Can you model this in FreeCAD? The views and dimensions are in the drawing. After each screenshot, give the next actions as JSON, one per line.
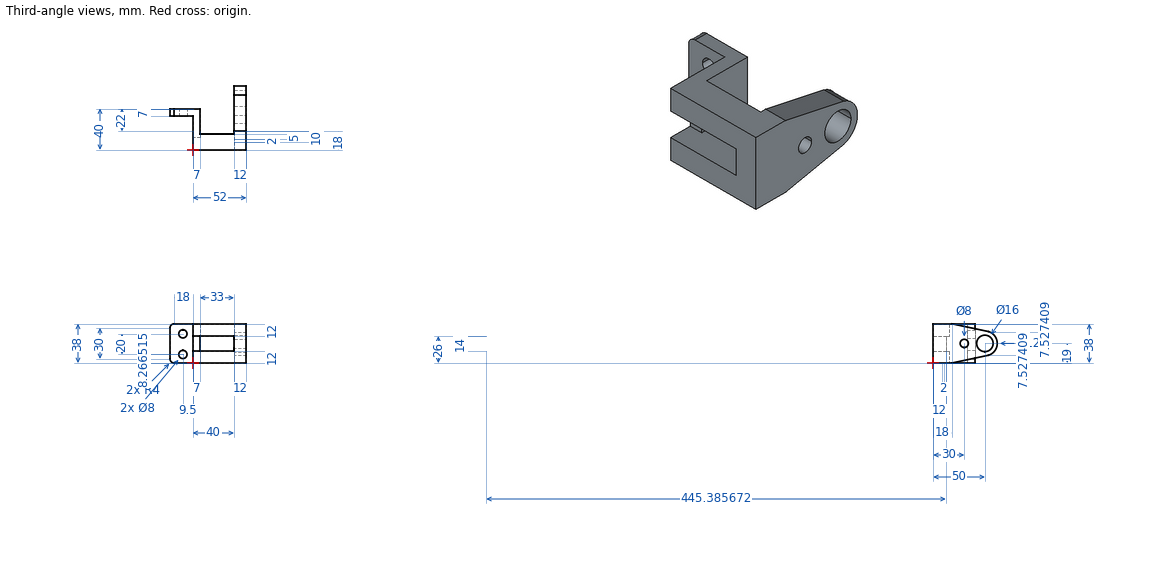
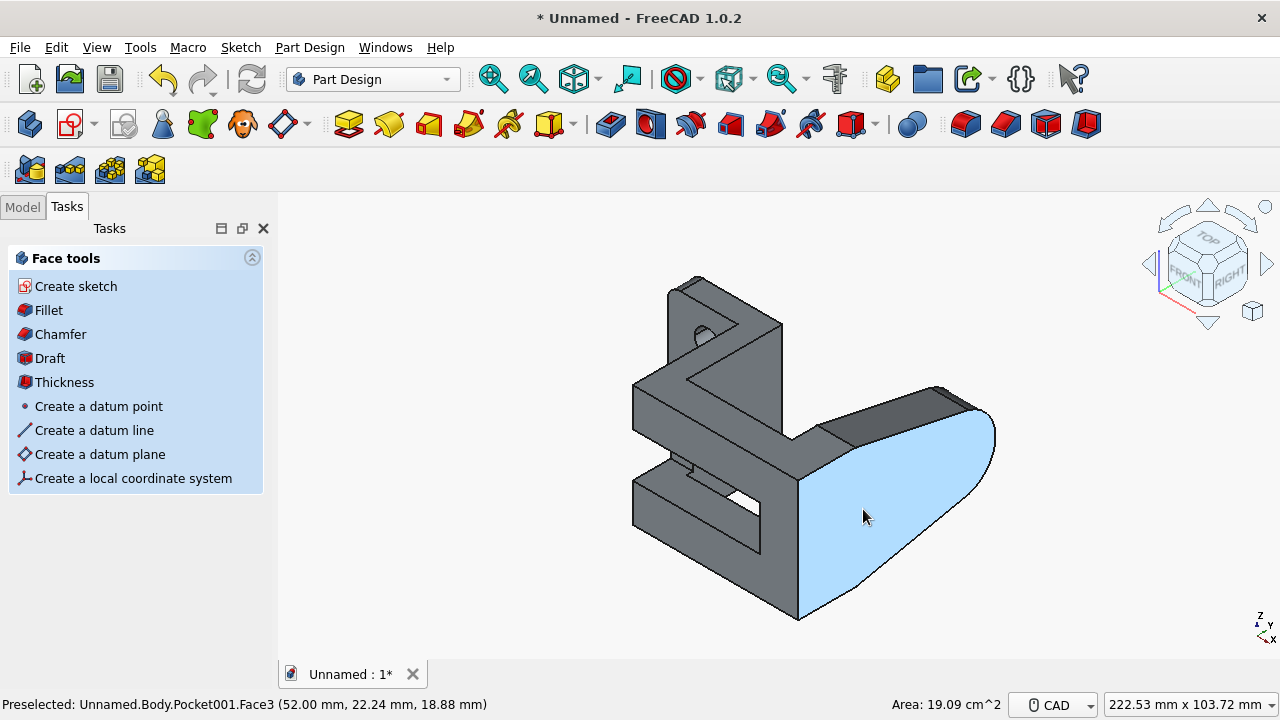
{"action": "left_click", "coordinate": [70, 124]}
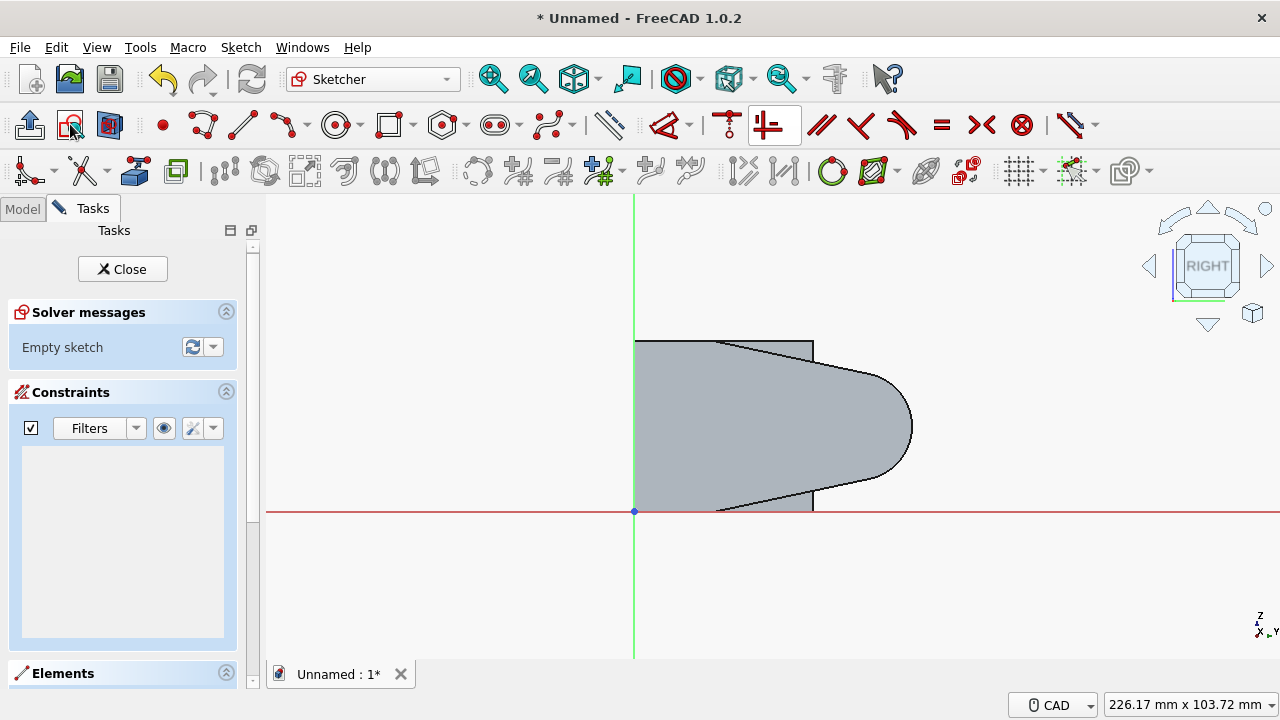
{"action": "scroll", "coordinate": [909, 426], "scroll_direction": "up", "scroll_amount": 7}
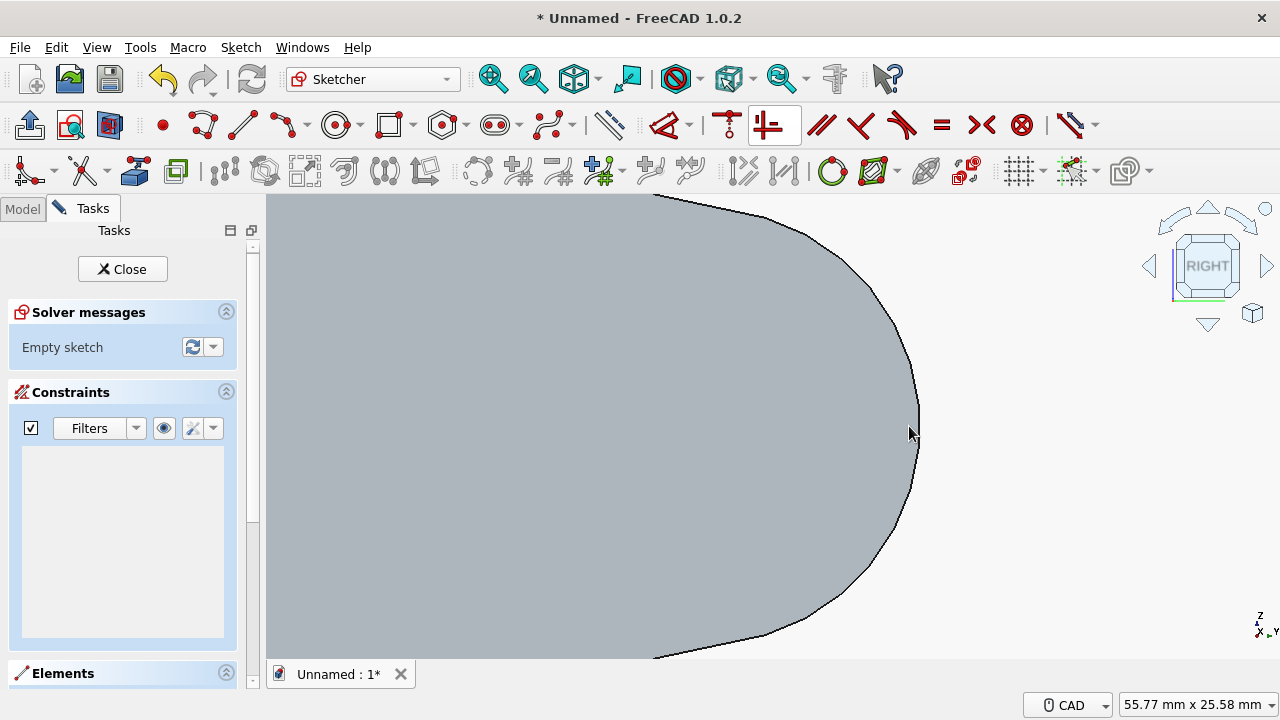
{"action": "left_click", "coordinate": [336, 126]}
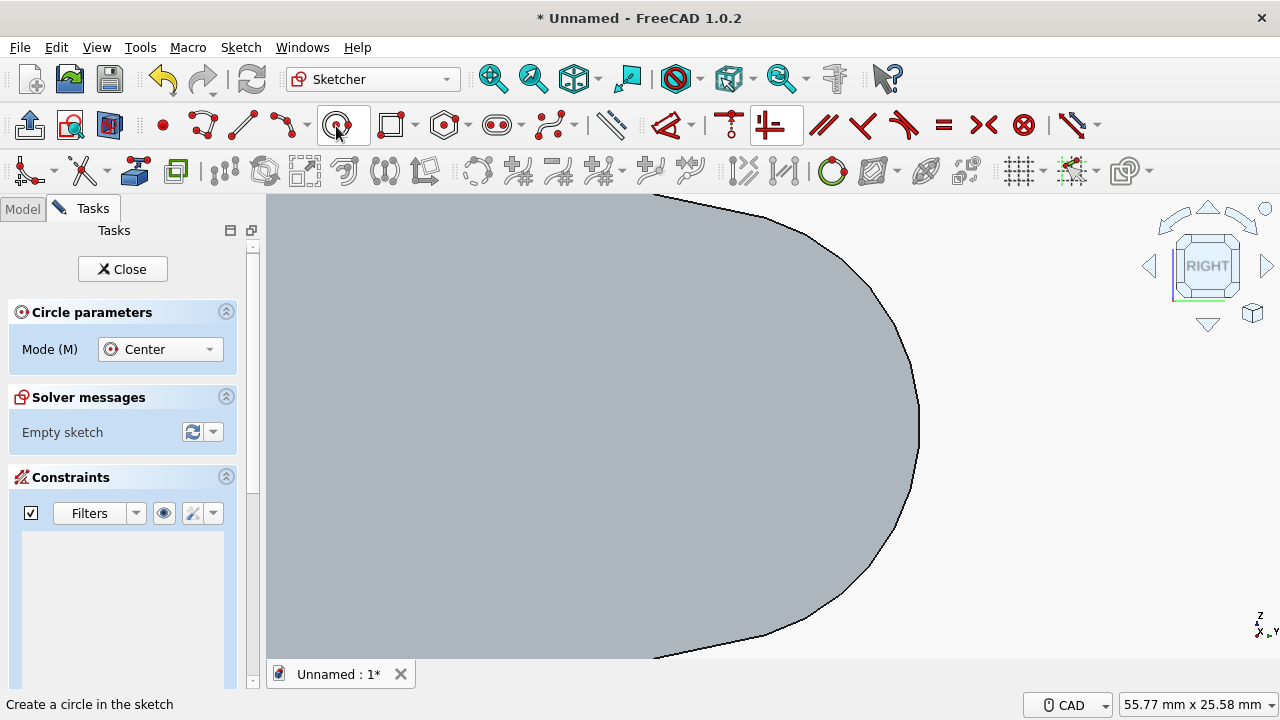
{"action": "left_click", "coordinate": [702, 426]}
{"action": "left_click", "coordinate": [804, 324]}
{"action": "key", "text": "Escape"}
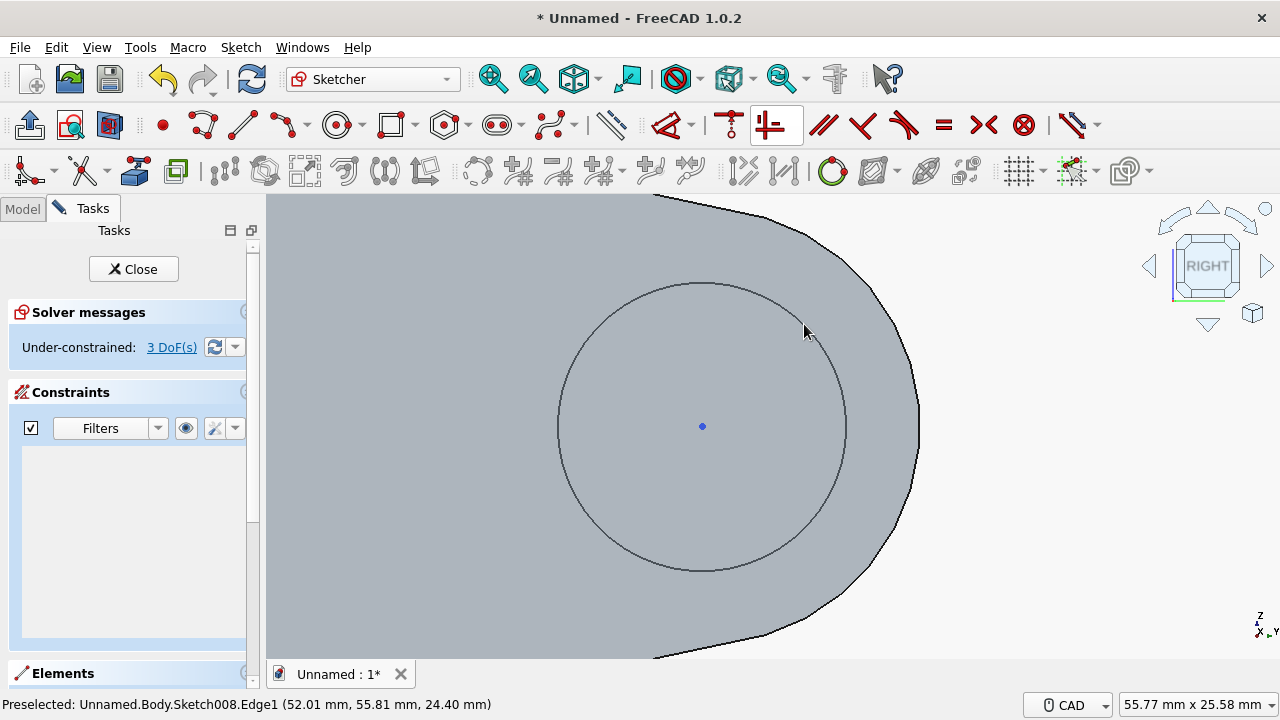
{"action": "left_click", "coordinate": [666, 126]}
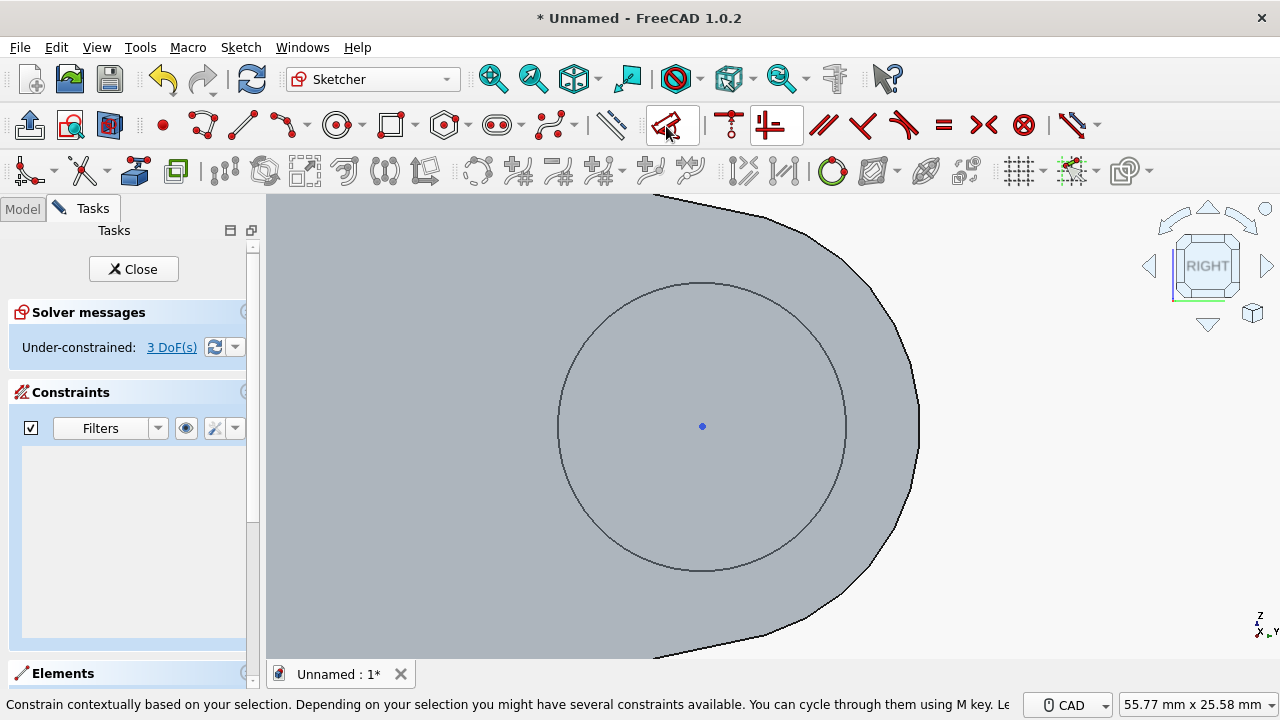
{"action": "left_click", "coordinate": [804, 325]}
{"action": "left_click", "coordinate": [827, 302]}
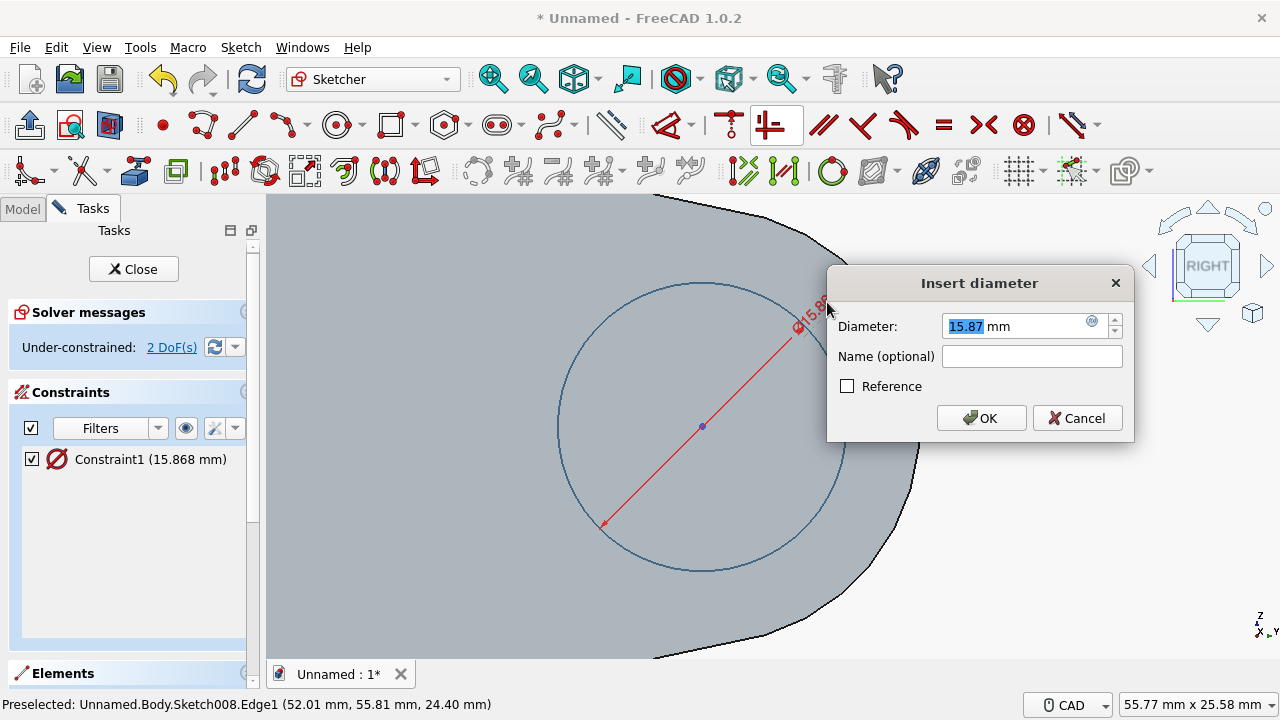
{"action": "type", "text": "16"}
{"action": "key", "text": "Return"}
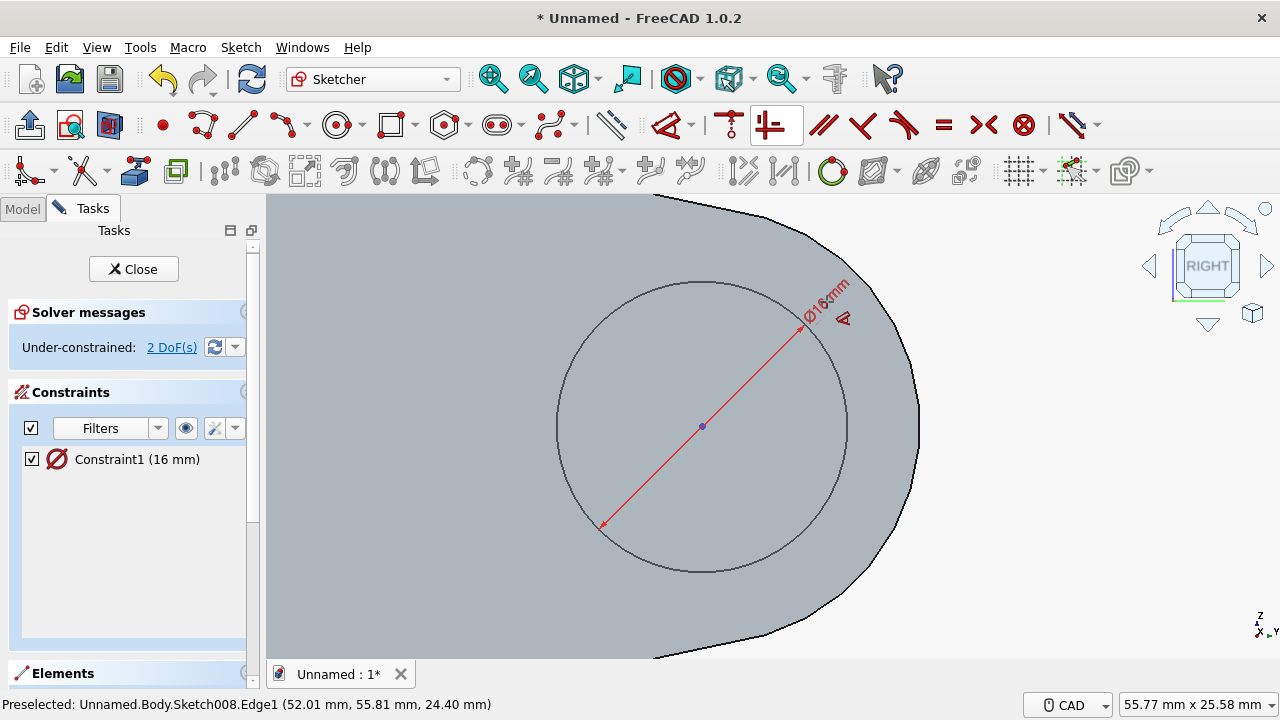
{"action": "left_click", "coordinate": [702, 427]}
{"action": "left_click", "coordinate": [498, 393]}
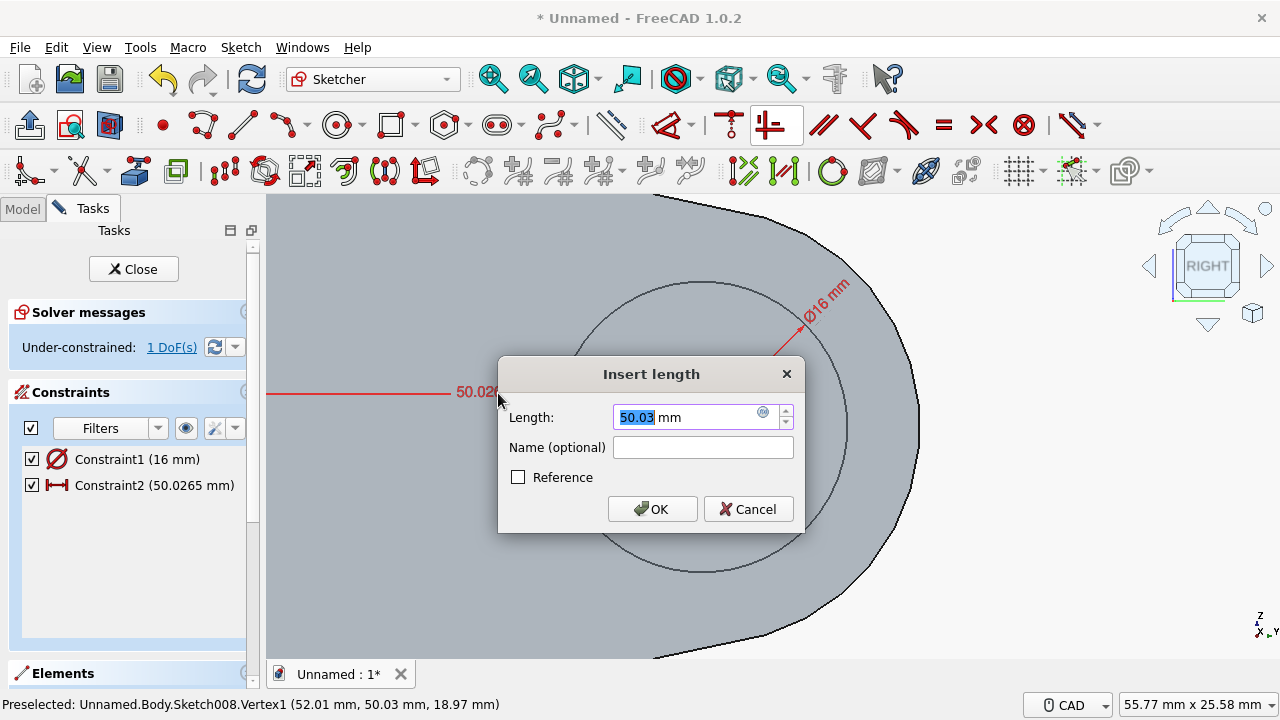
{"action": "type", "text": "50"}
{"action": "key", "text": "Return"}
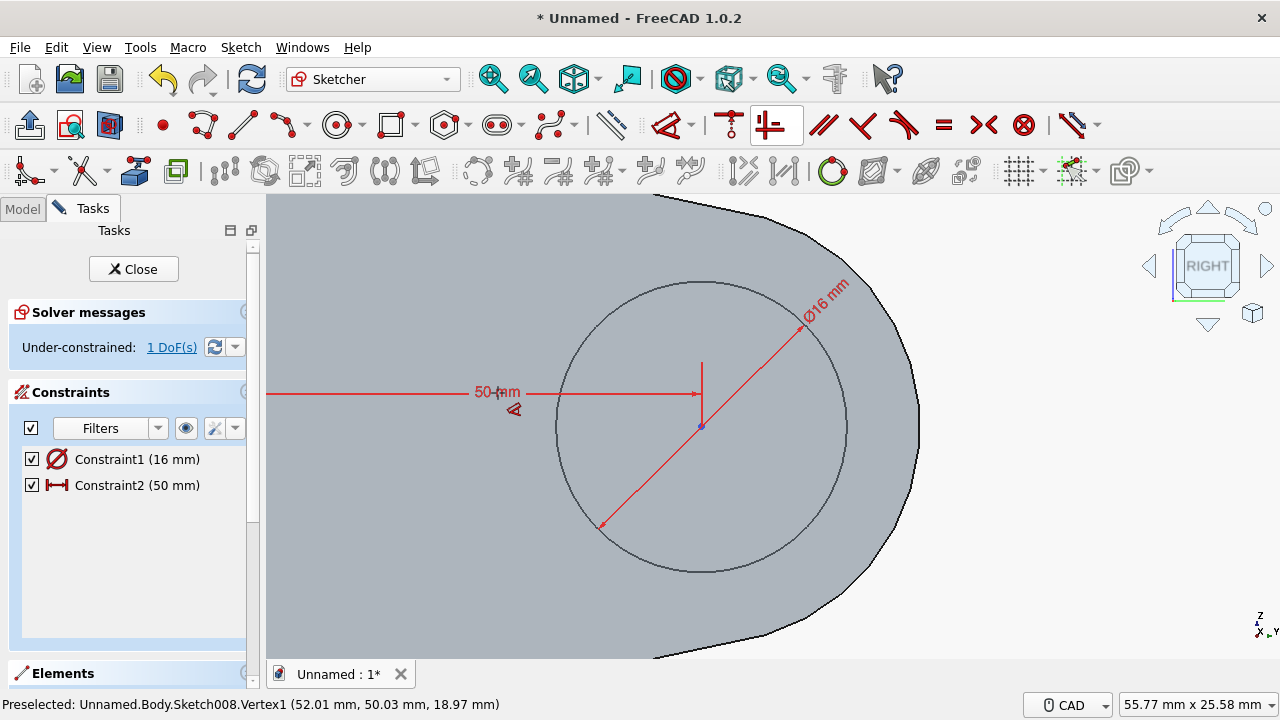
{"action": "left_click", "coordinate": [702, 427]}
{"action": "left_click", "coordinate": [736, 529]}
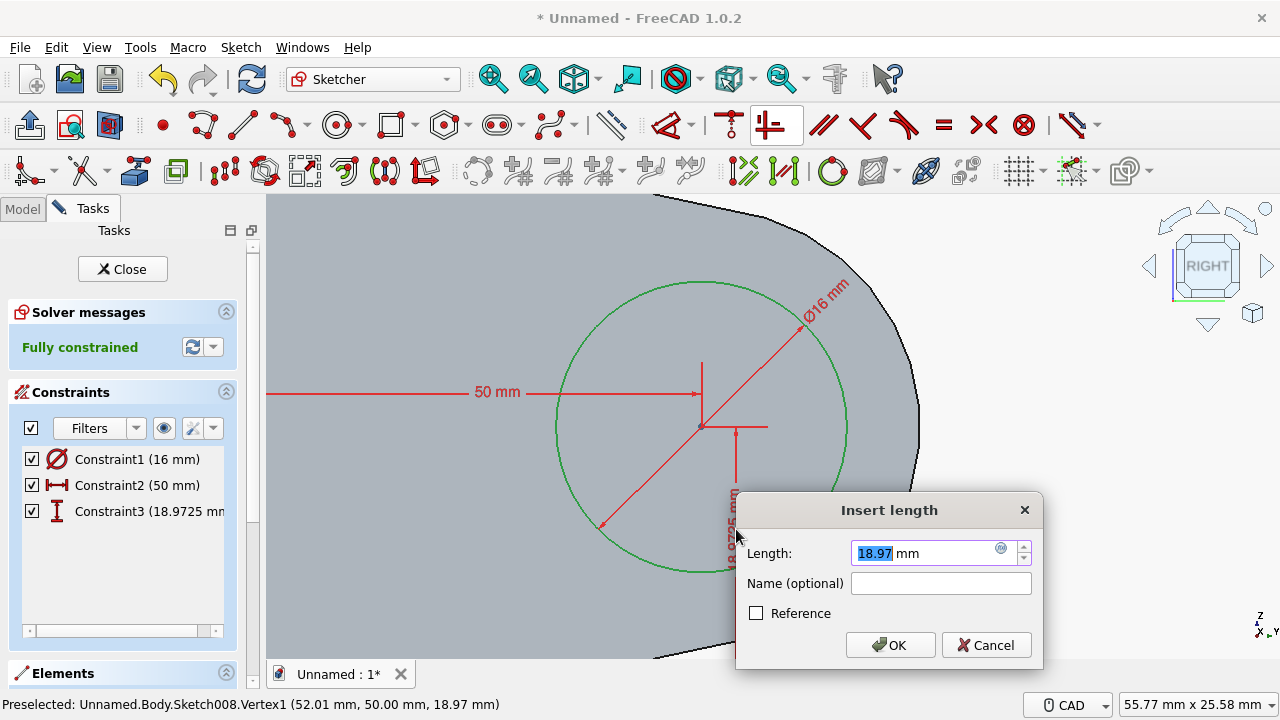
{"action": "type", "text": "19"}
{"action": "key", "text": "Return"}
{"action": "key", "text": "Escape"}